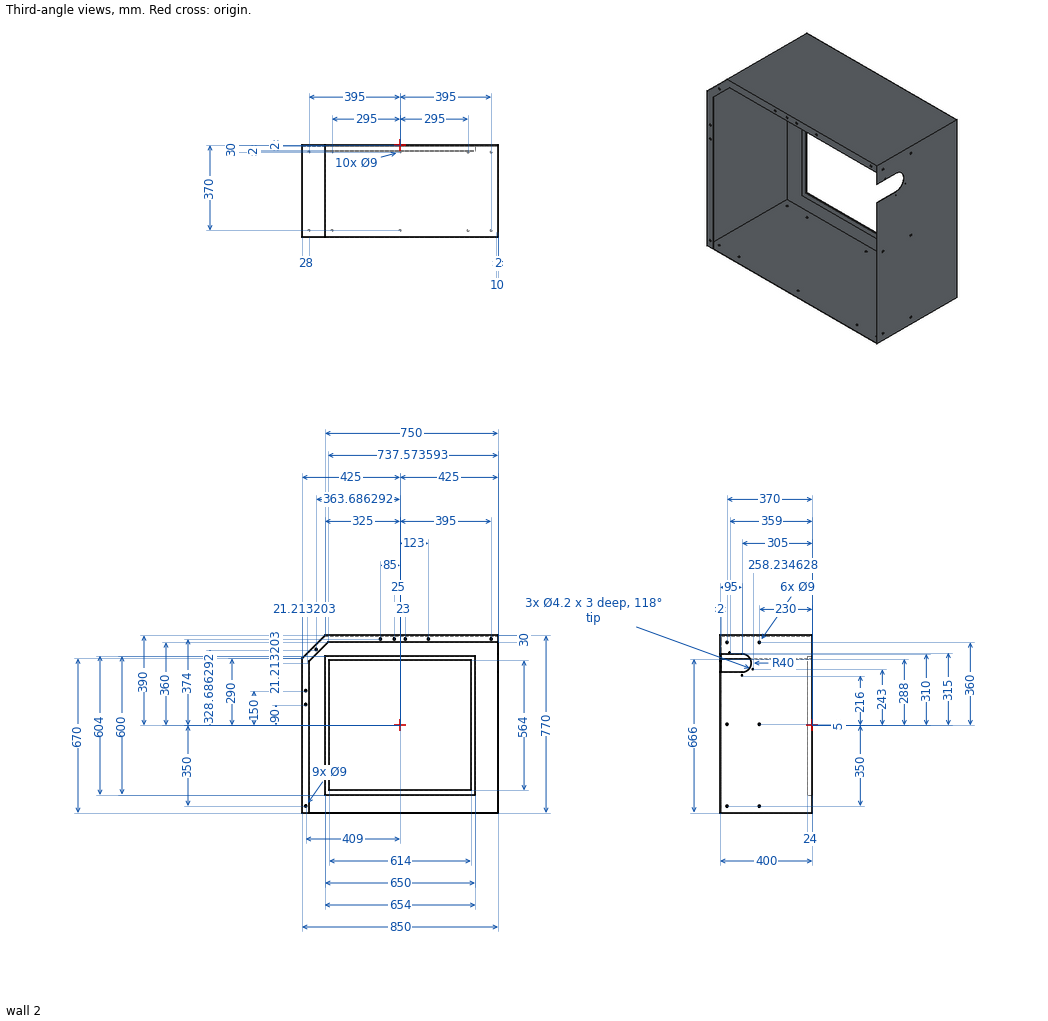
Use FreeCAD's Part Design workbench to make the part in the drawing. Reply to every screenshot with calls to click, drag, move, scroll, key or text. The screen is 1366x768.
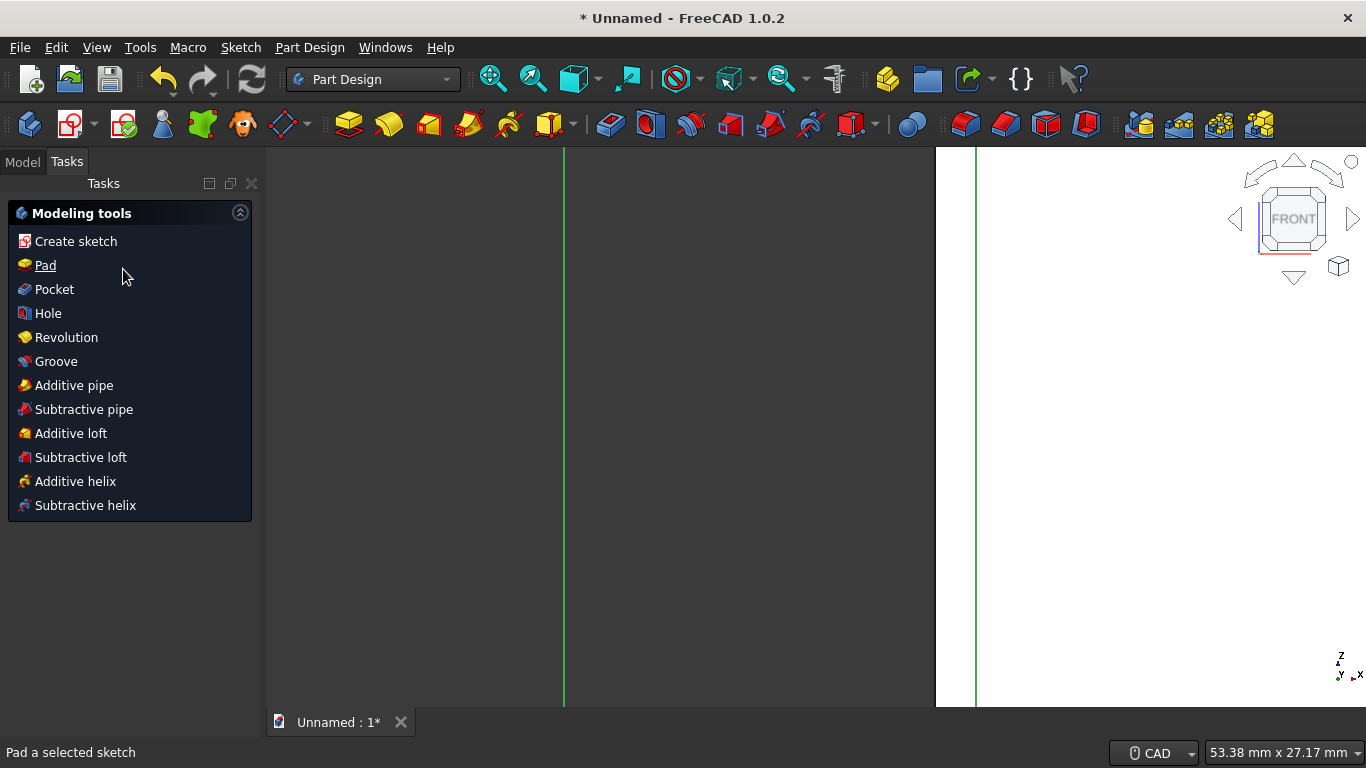
click(350, 124)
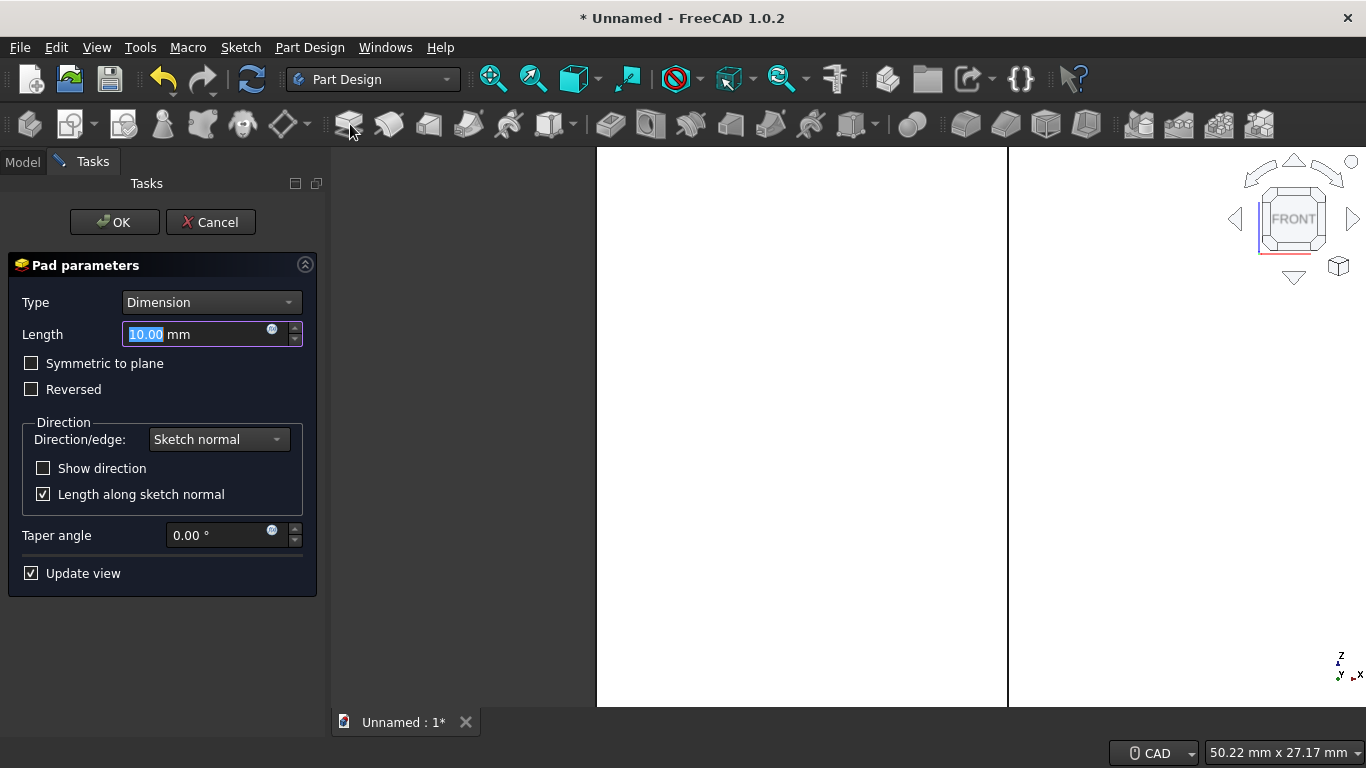
text(2)
key(Tab)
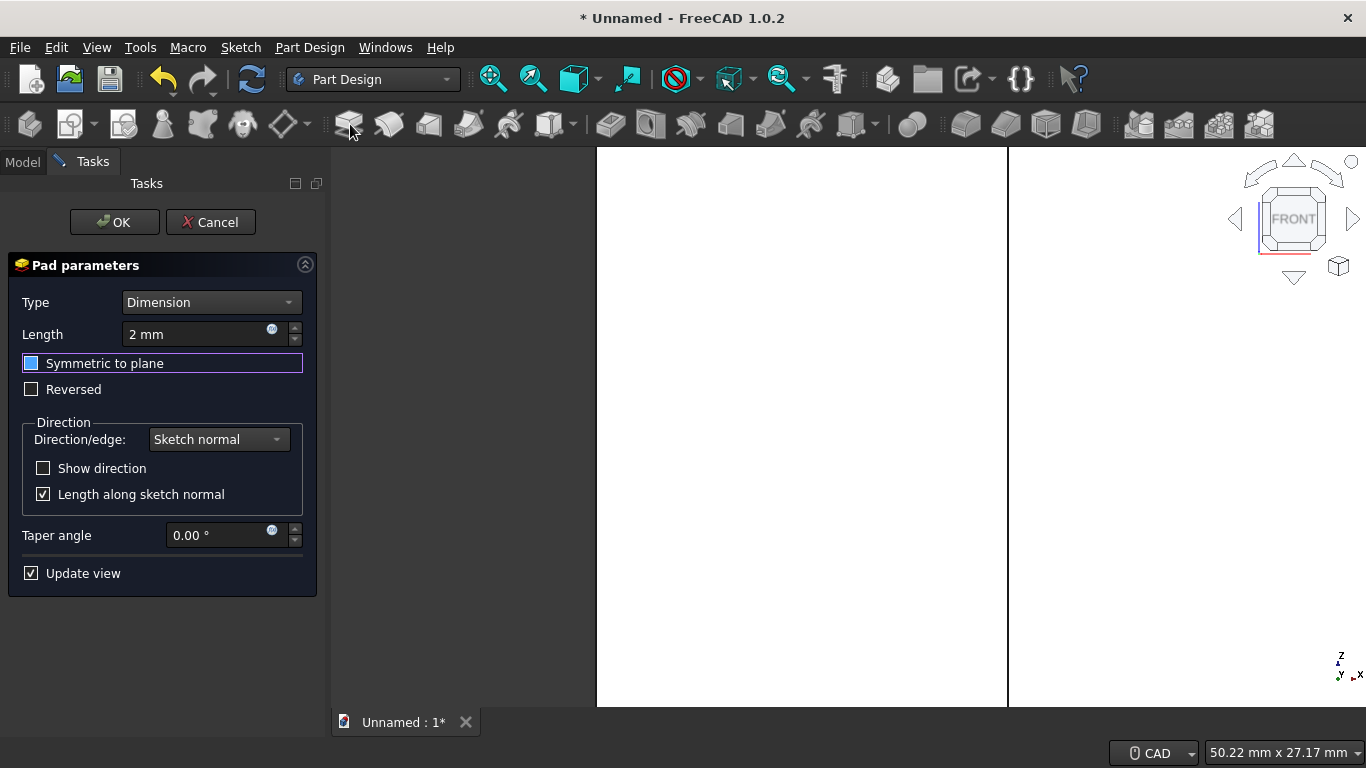
click(30, 389)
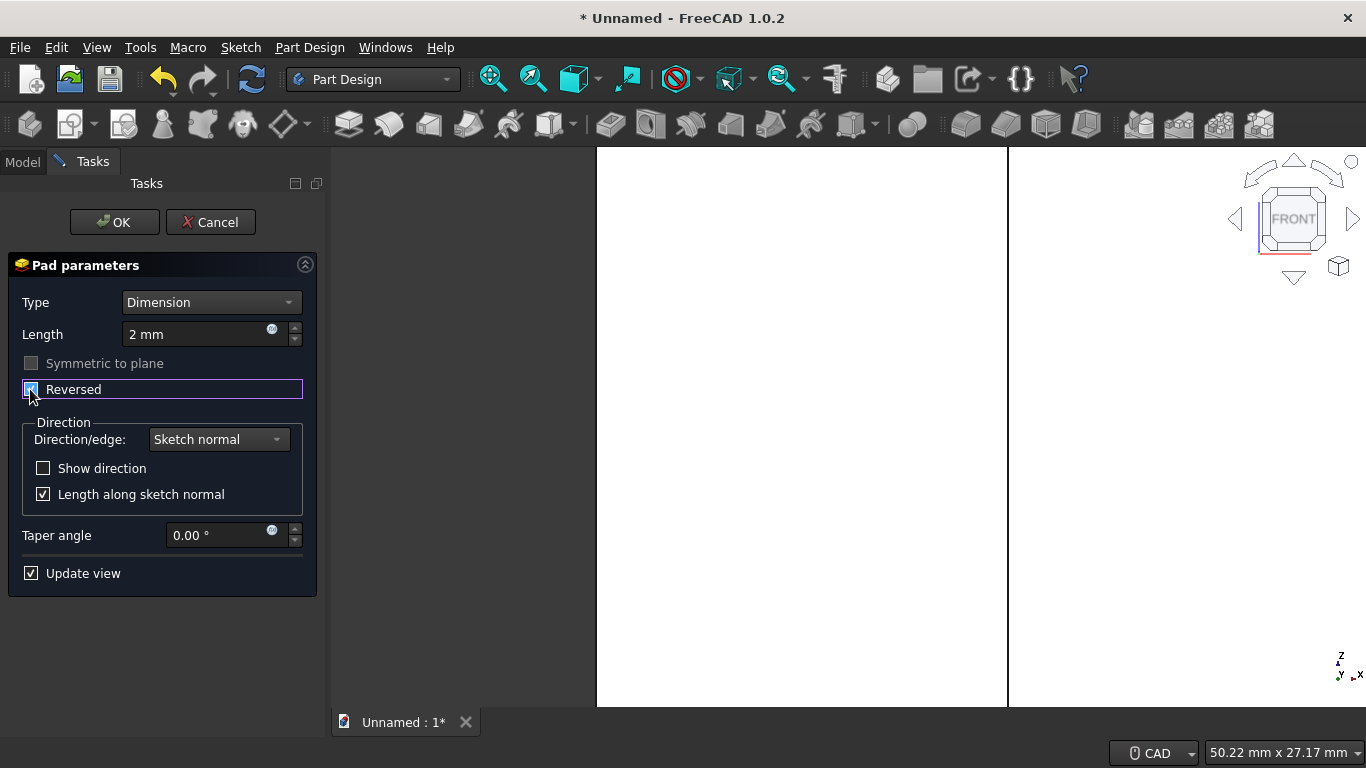
click(115, 222)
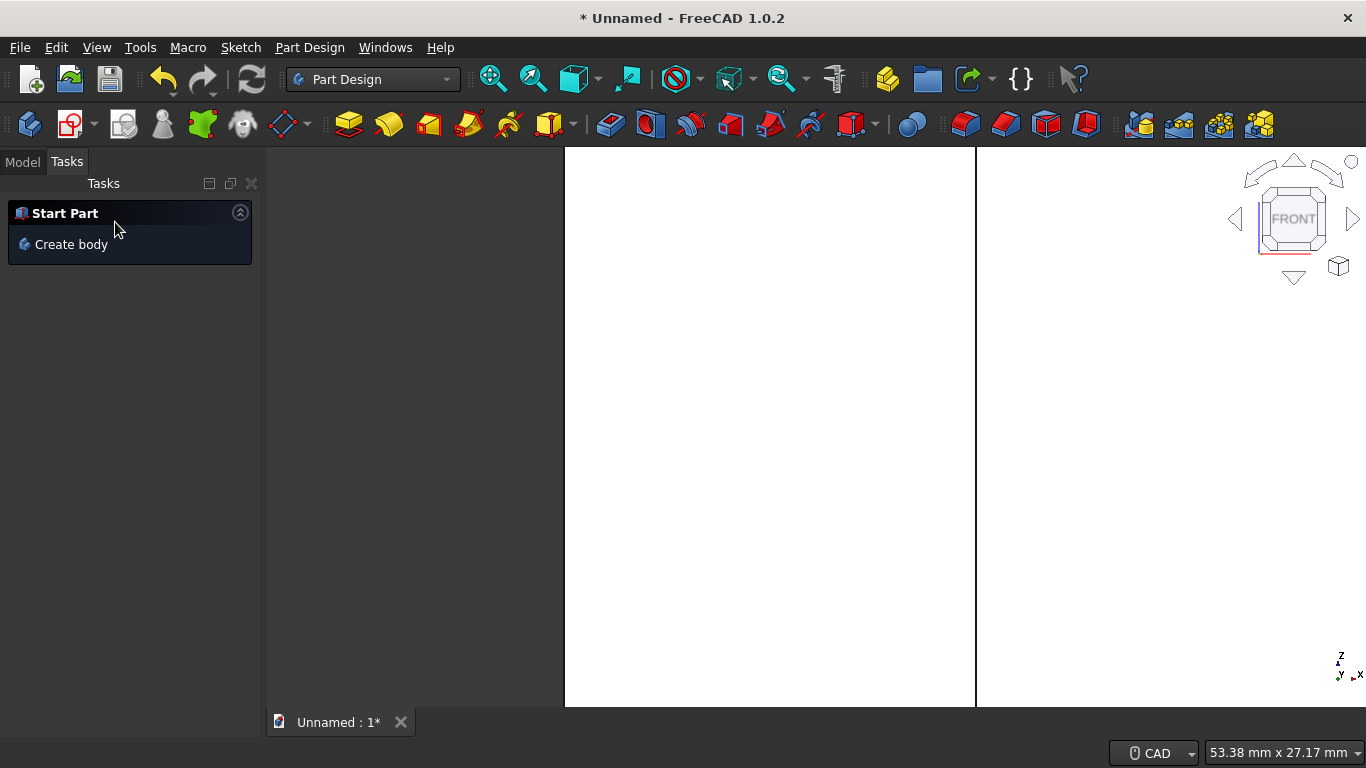
click(494, 80)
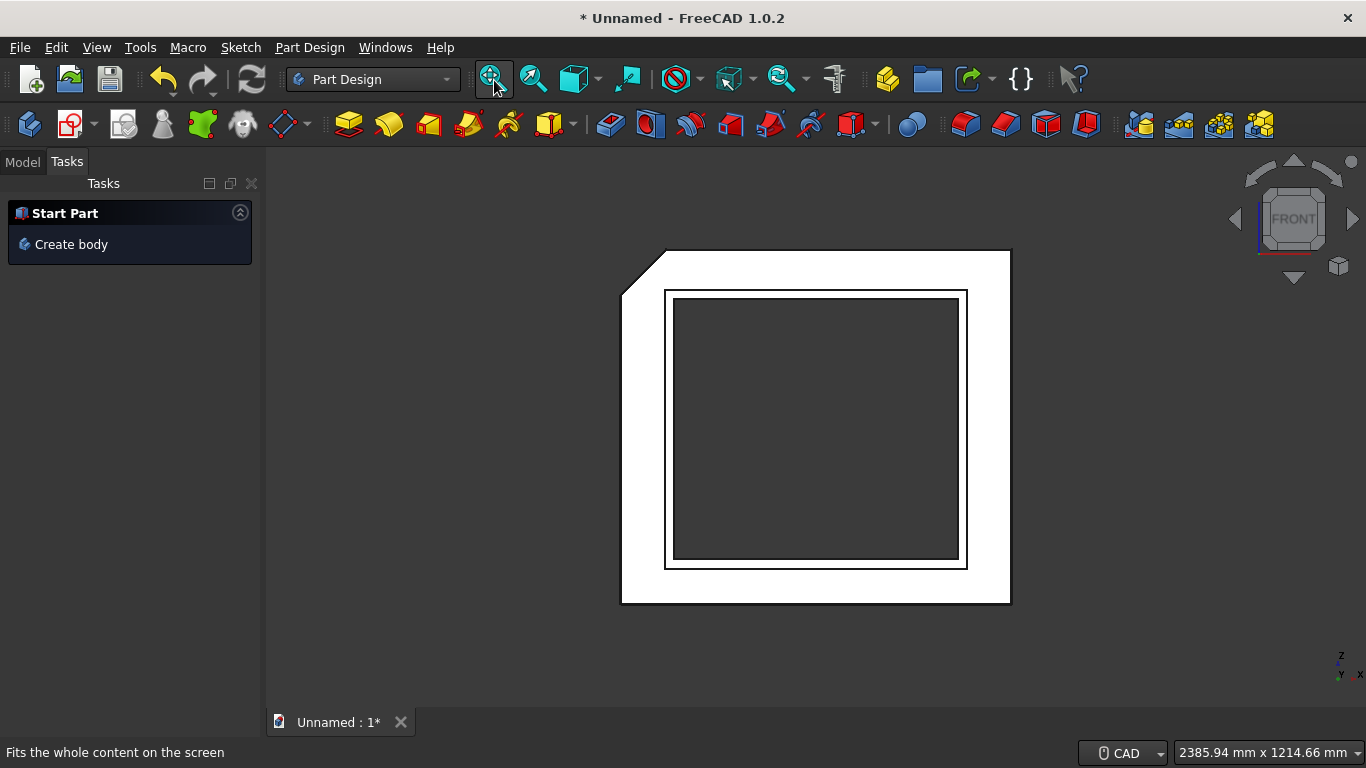
scroll(621, 397, up, 15)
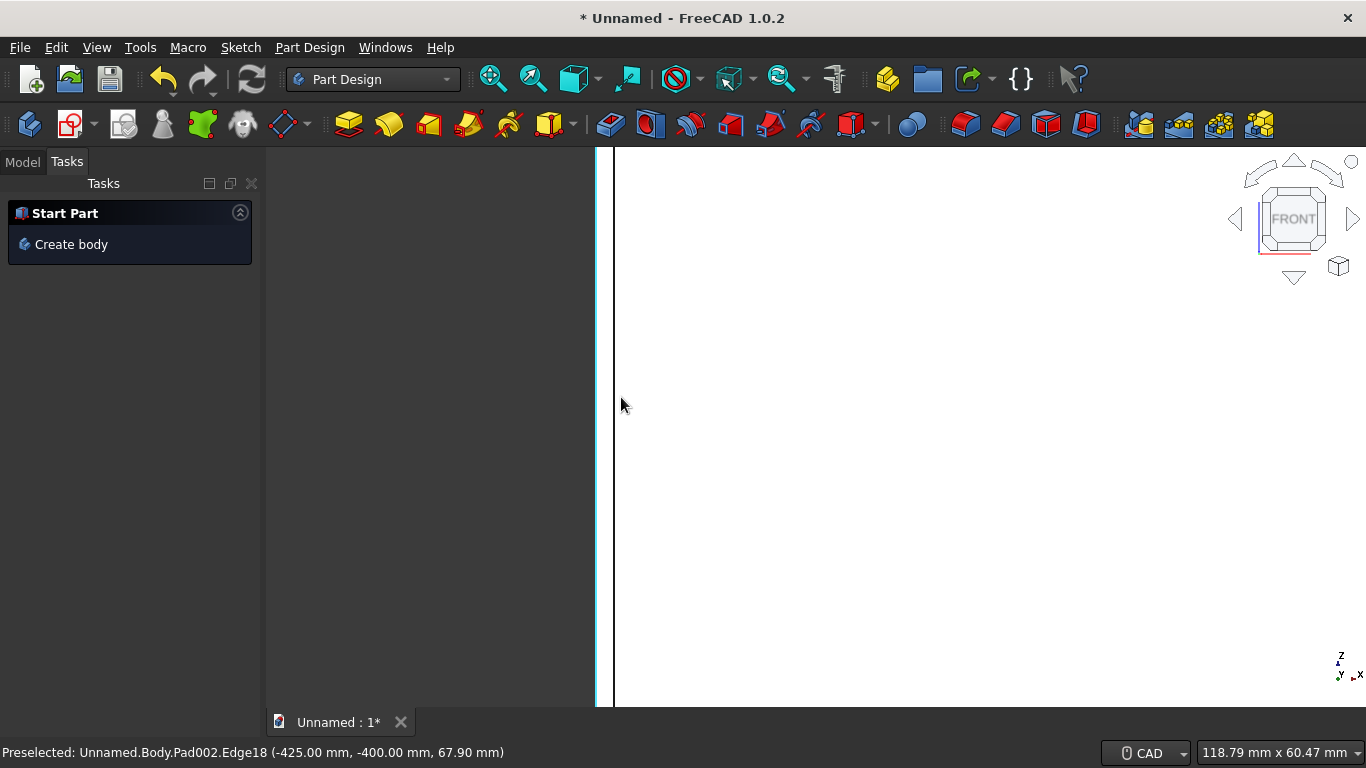
scroll(608, 415, up, 4)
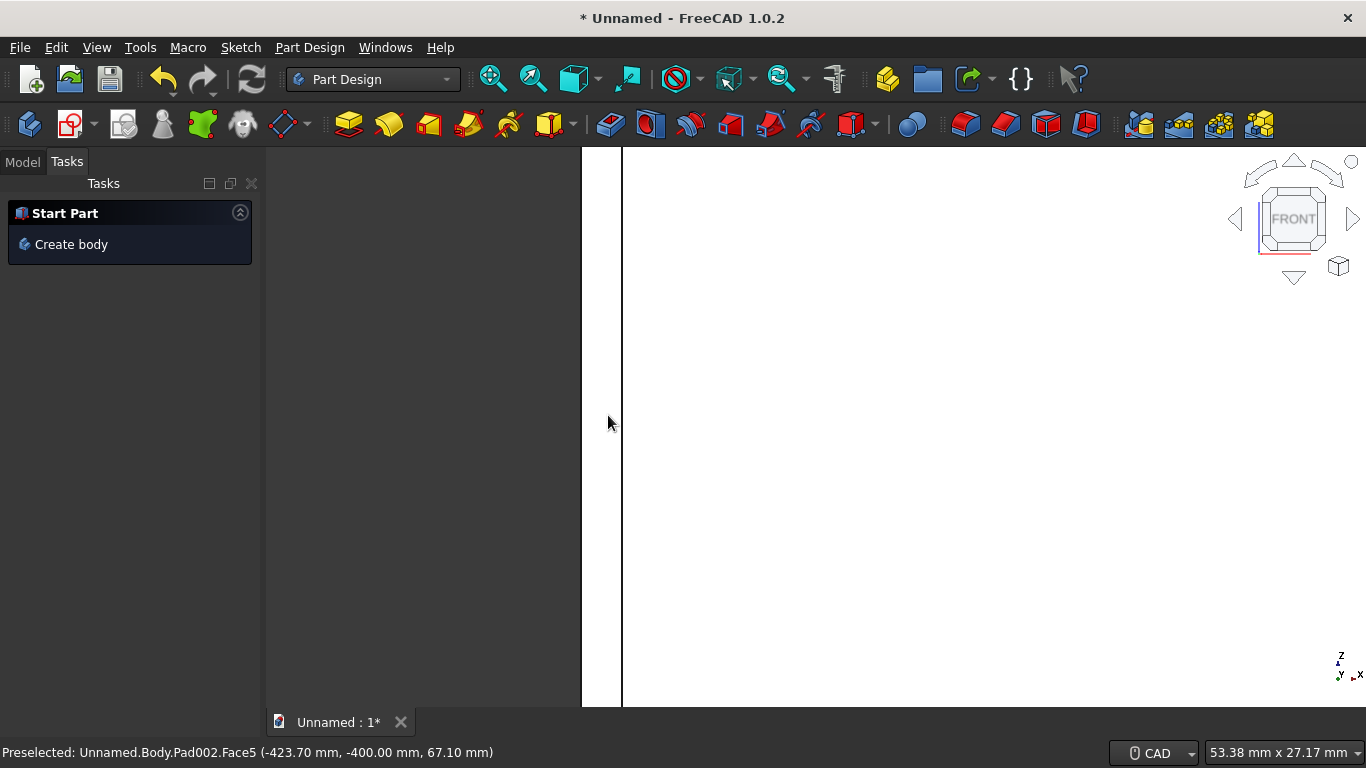
click(608, 416)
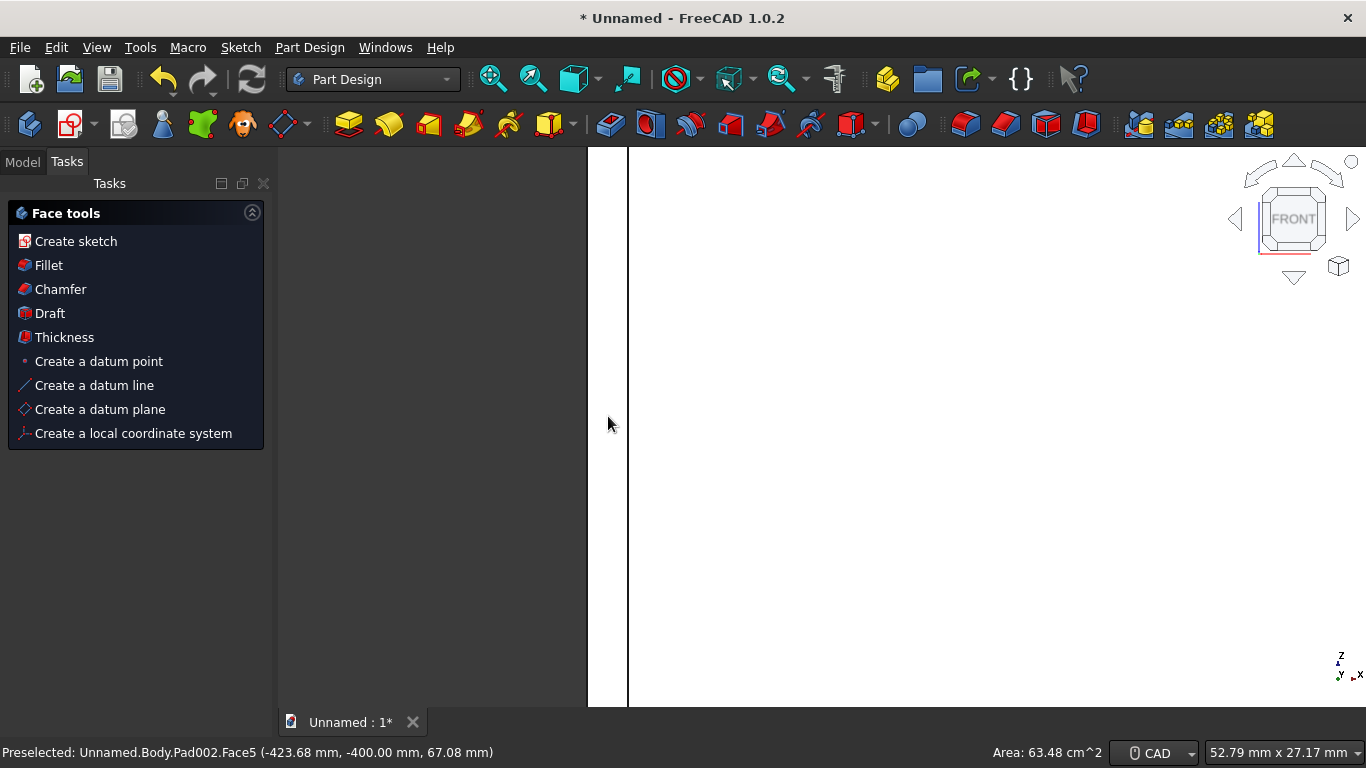
click(70, 124)